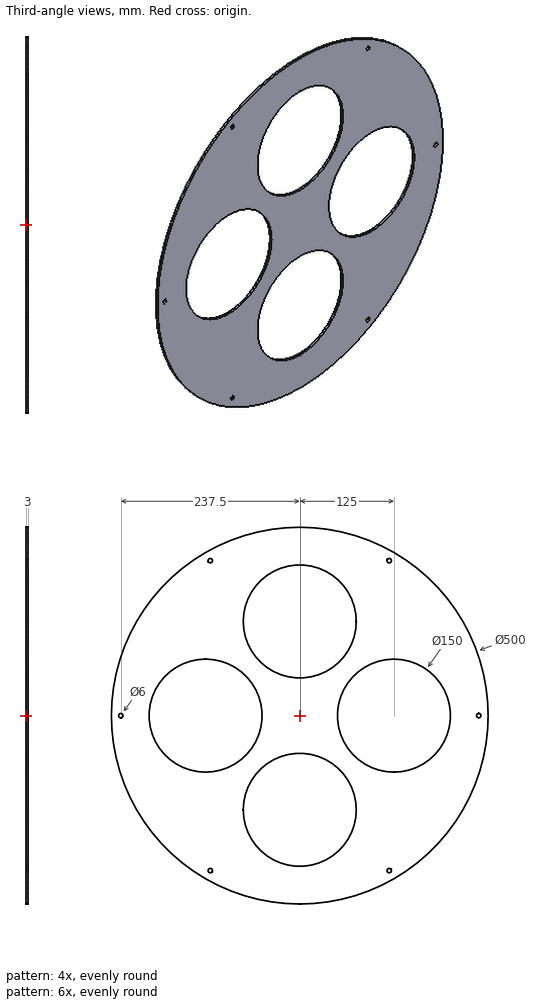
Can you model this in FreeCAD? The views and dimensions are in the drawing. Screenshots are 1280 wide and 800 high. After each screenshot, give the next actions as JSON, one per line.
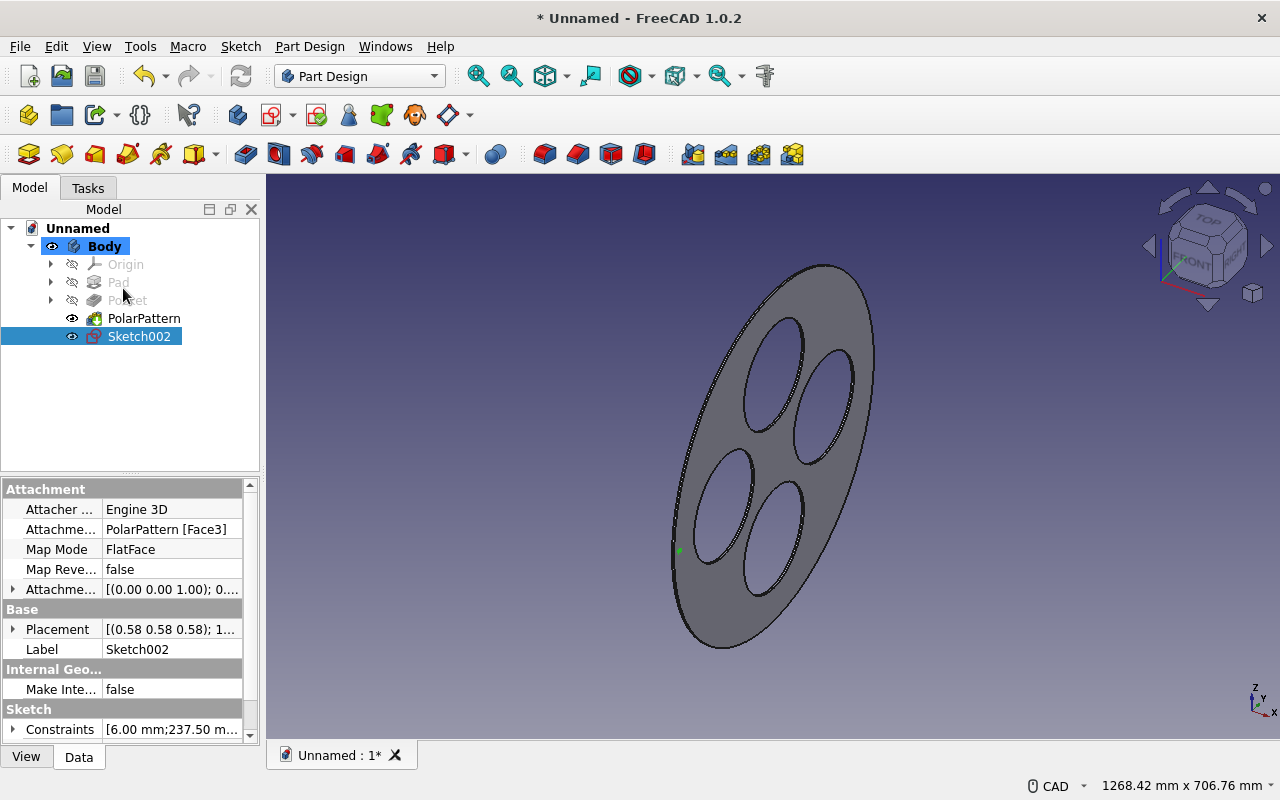
{"action": "left_click", "coordinate": [246, 154]}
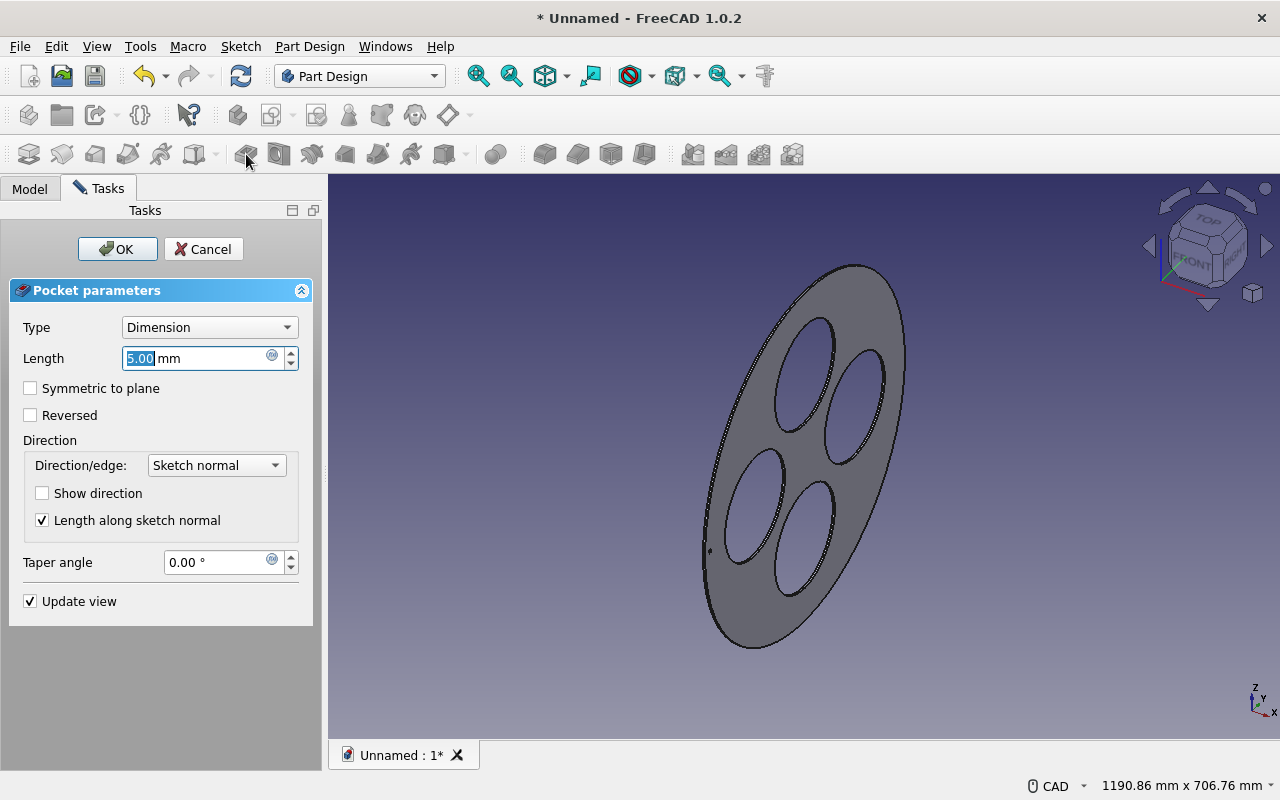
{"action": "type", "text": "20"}
{"action": "key", "text": "Tab"}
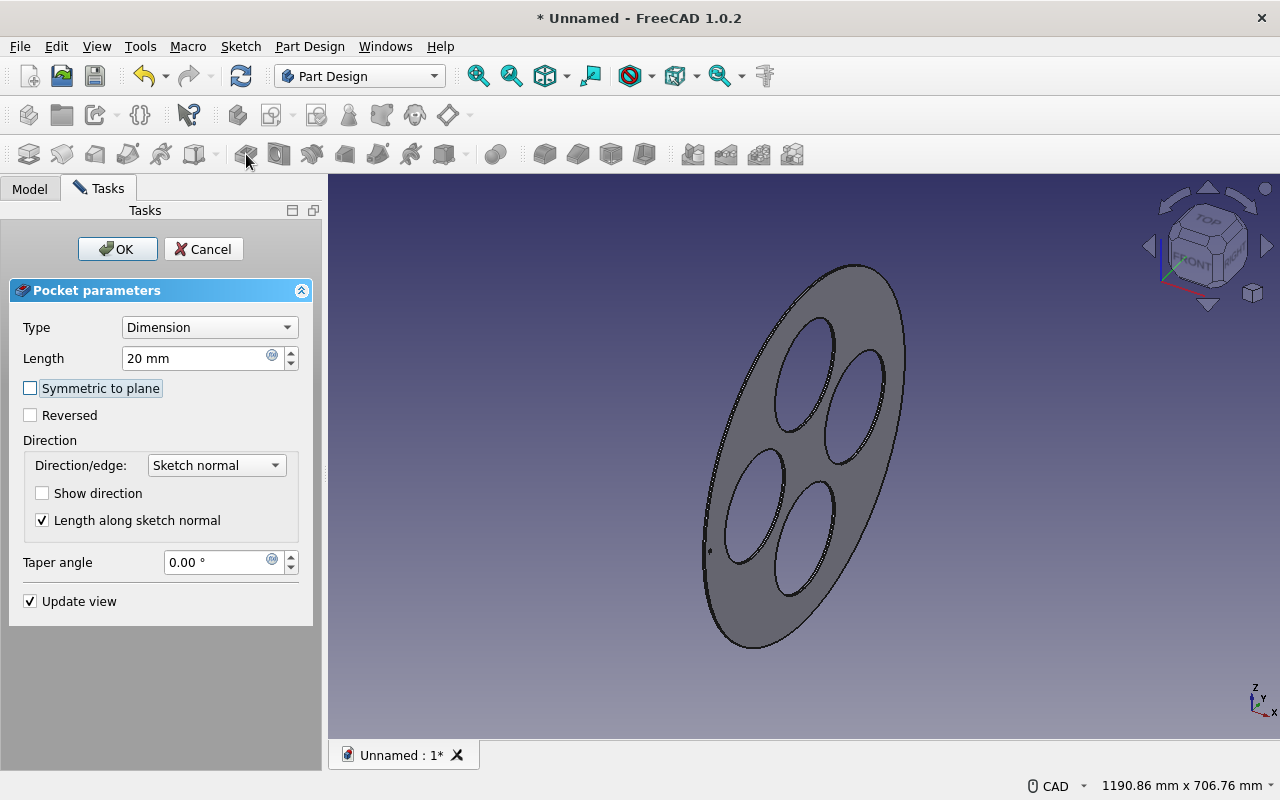
{"action": "left_click", "coordinate": [118, 249]}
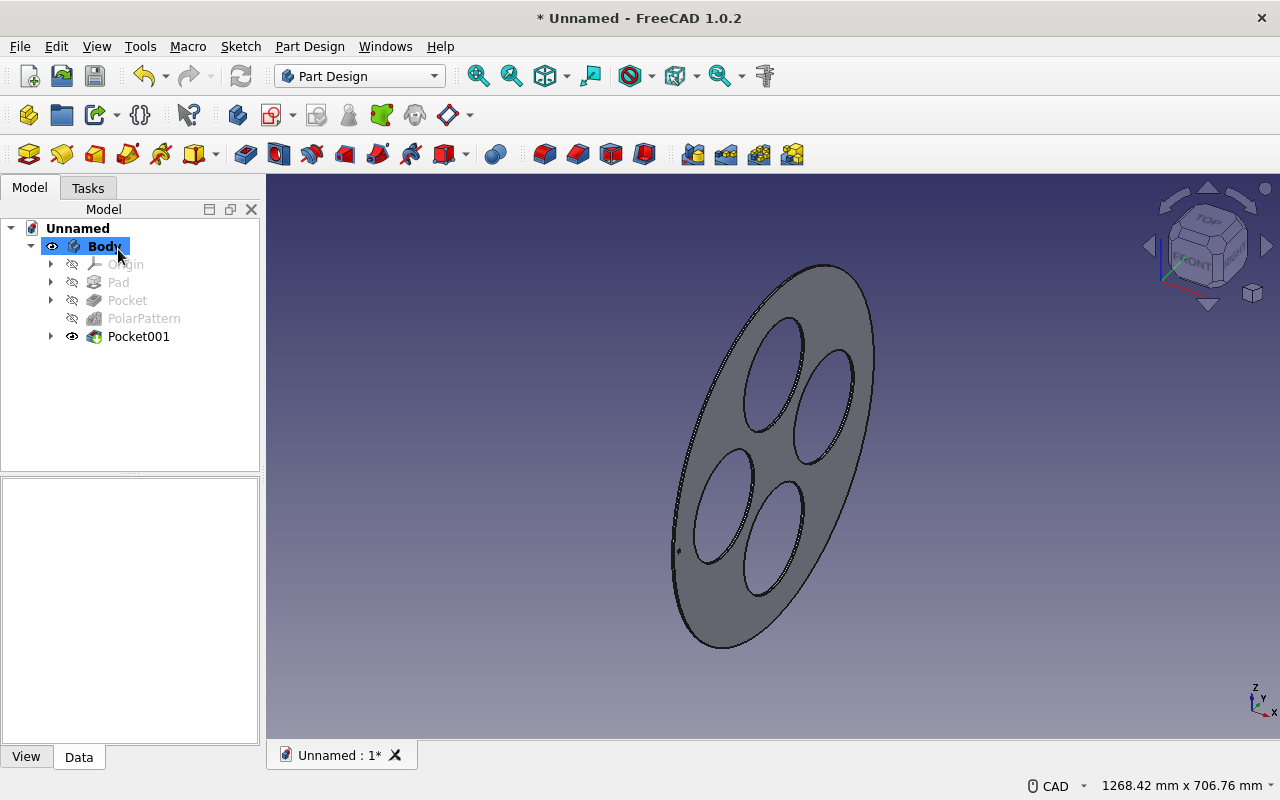
{"action": "left_click", "coordinate": [117, 336]}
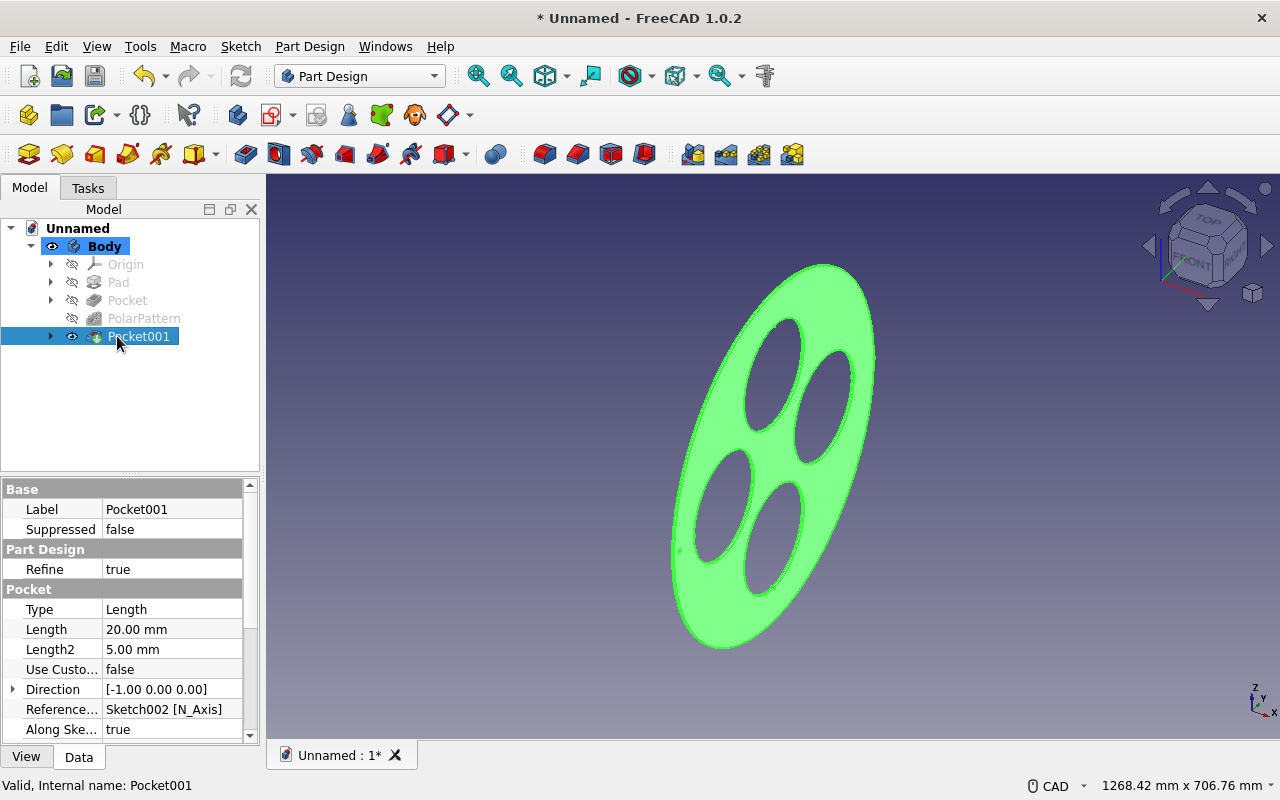
{"action": "left_click", "coordinate": [759, 154]}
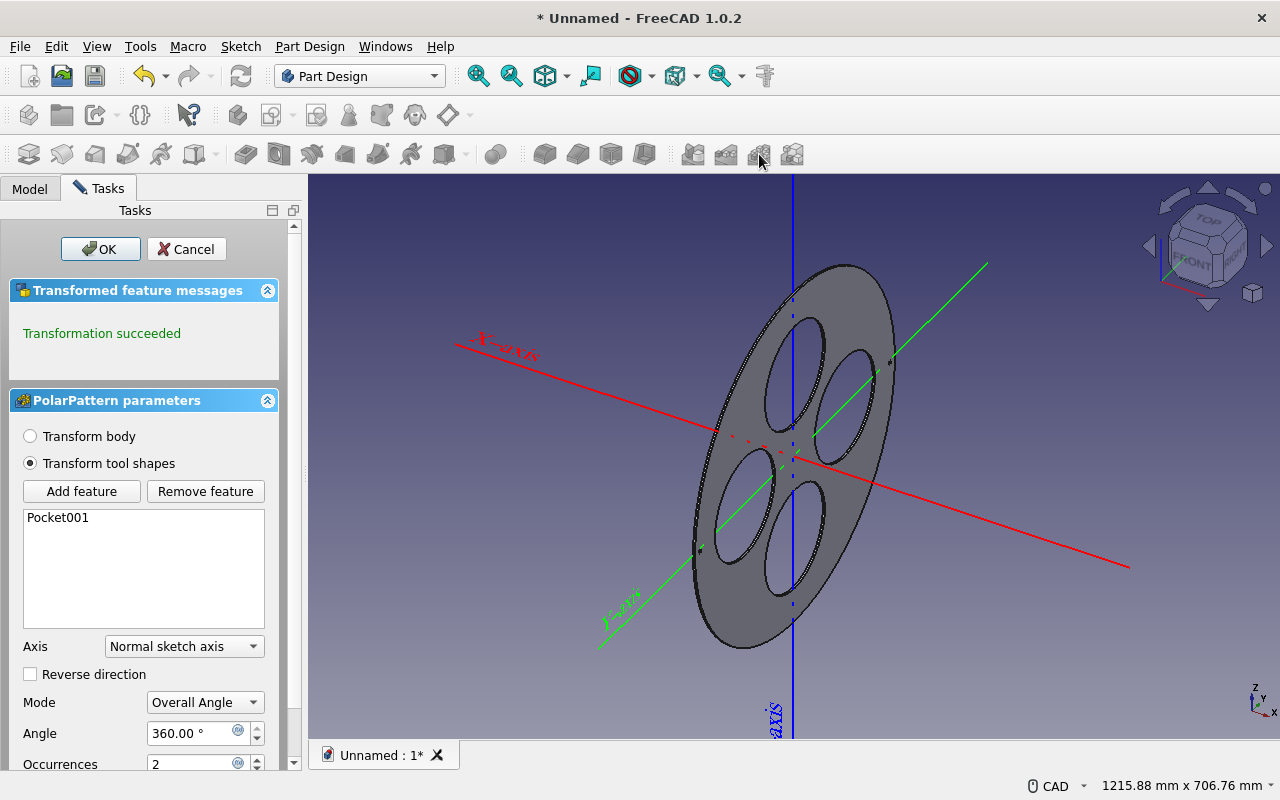
{"action": "left_click", "coordinate": [185, 646]}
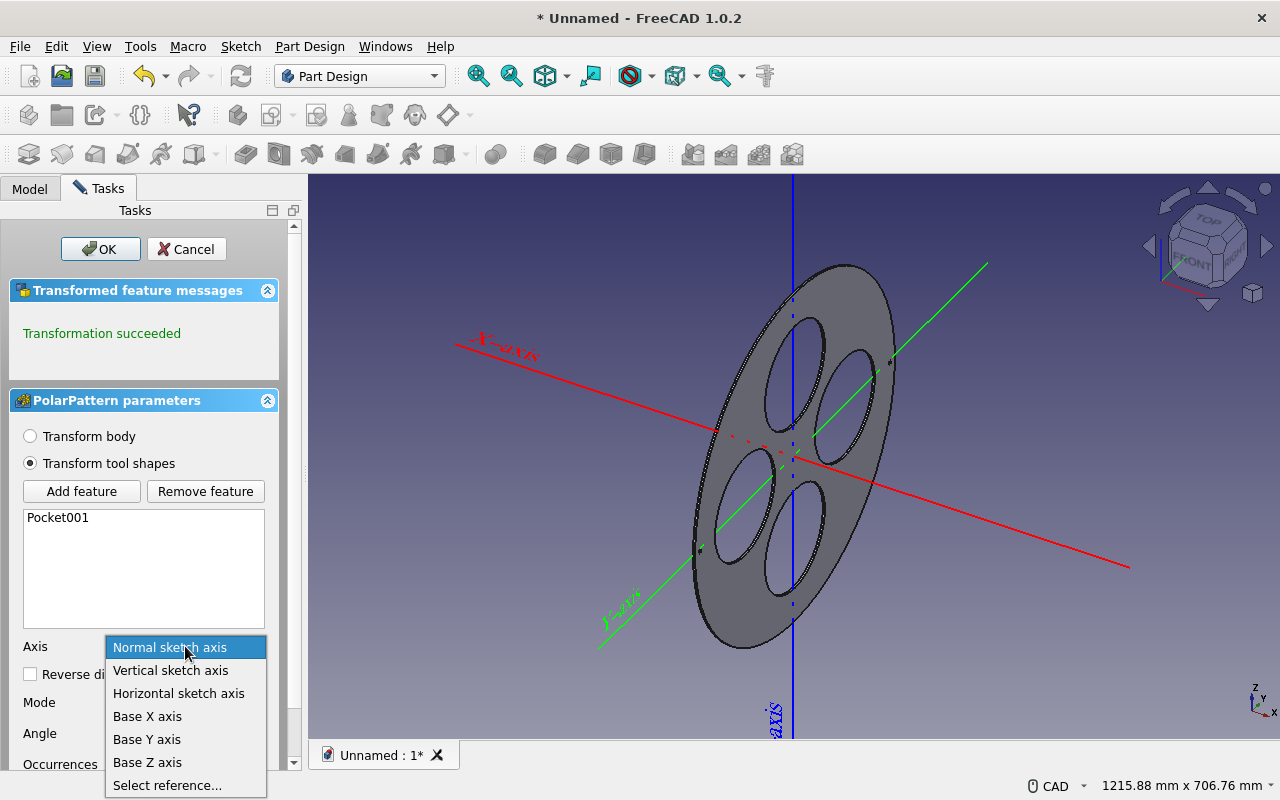
{"action": "left_click", "coordinate": [184, 716]}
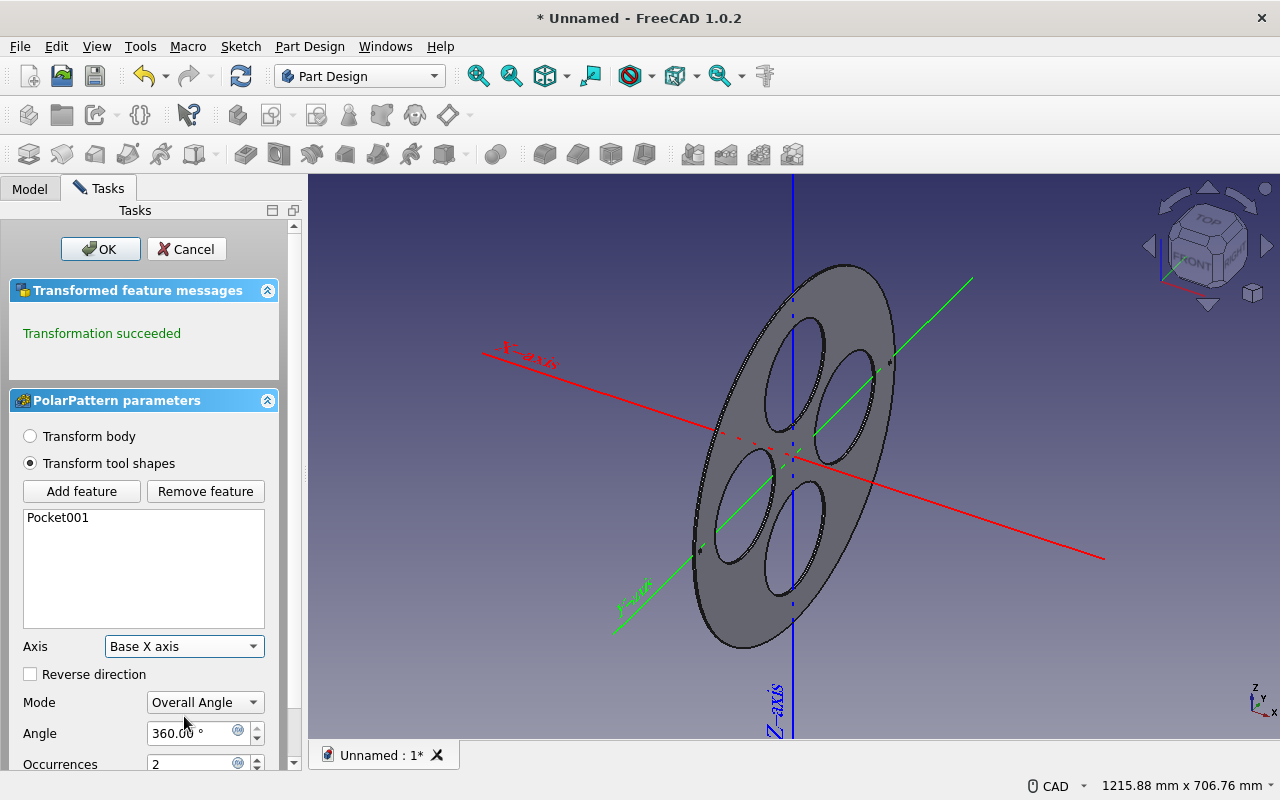
{"action": "scroll", "coordinate": [294, 495], "scroll_direction": "down", "scroll_amount": 2}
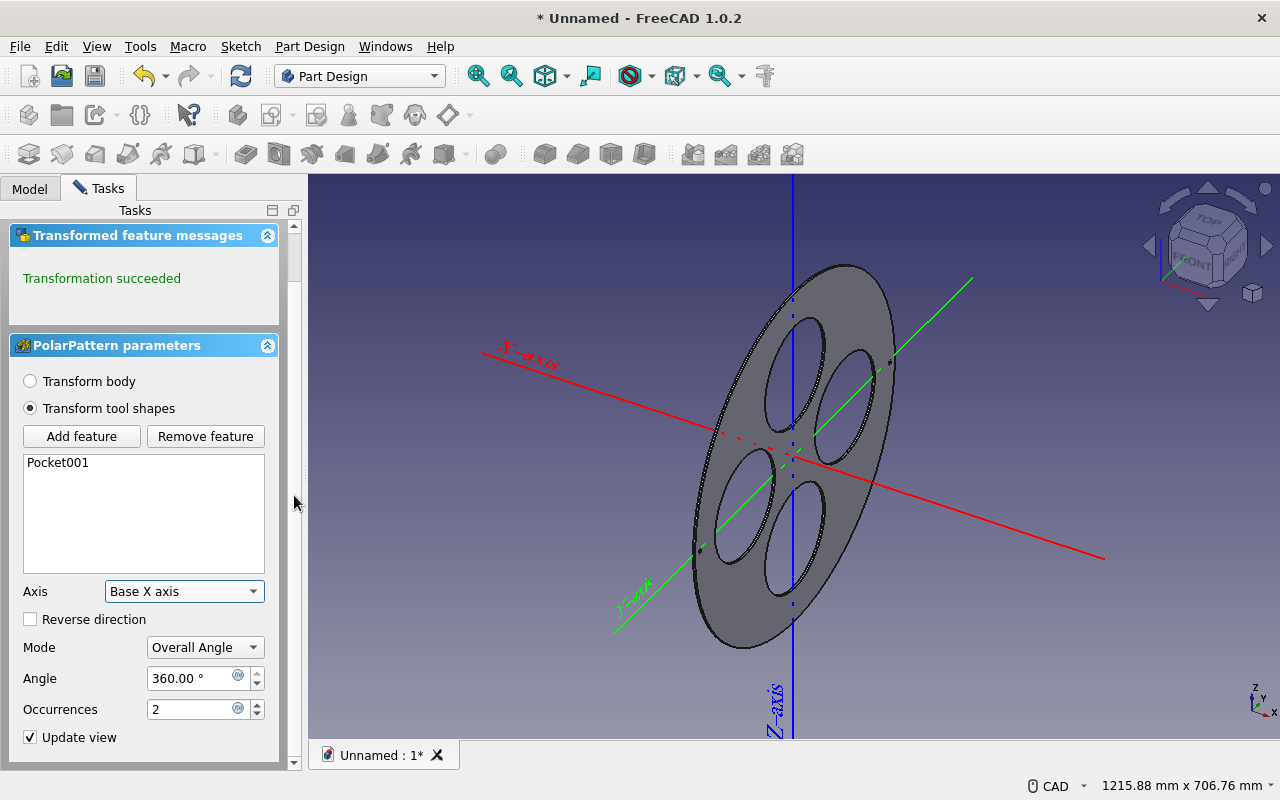
{"action": "triple_click", "coordinate": [199, 710]}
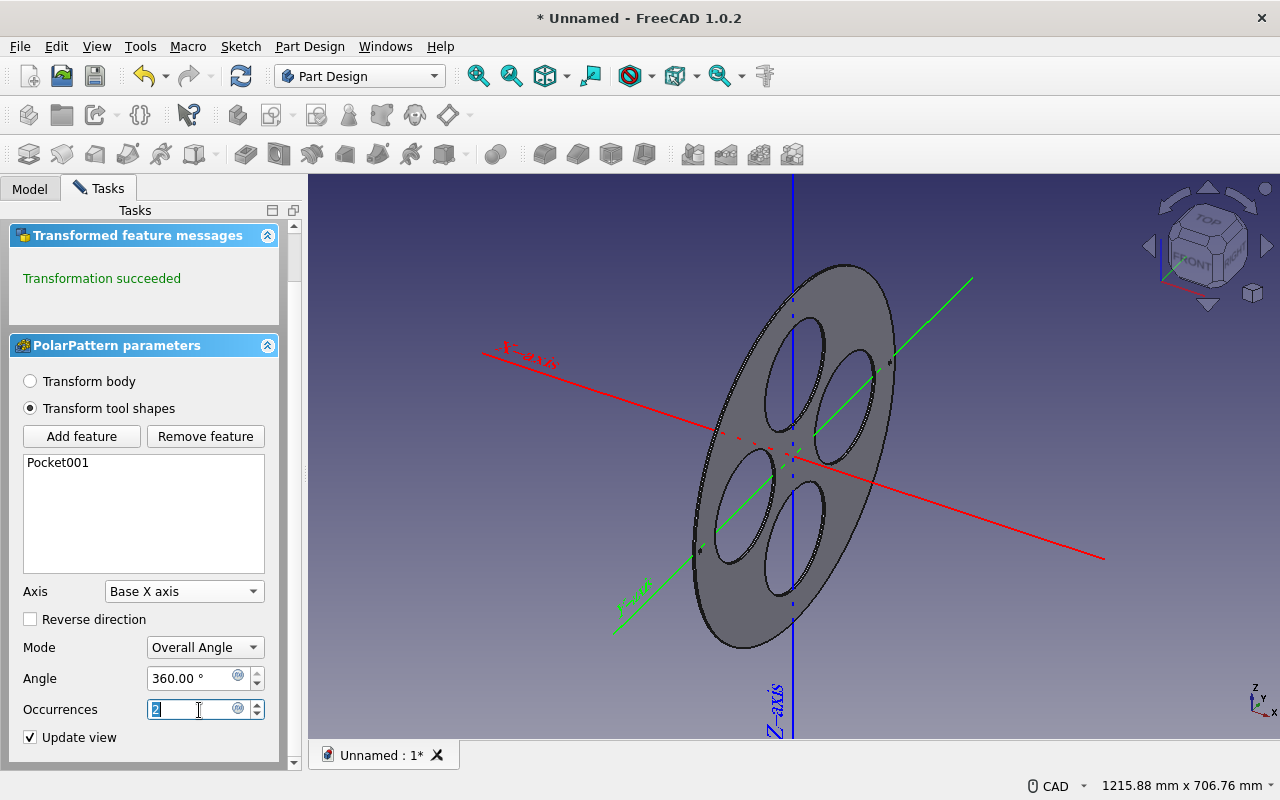
{"action": "type", "text": "6"}
{"action": "key", "text": "Tab"}